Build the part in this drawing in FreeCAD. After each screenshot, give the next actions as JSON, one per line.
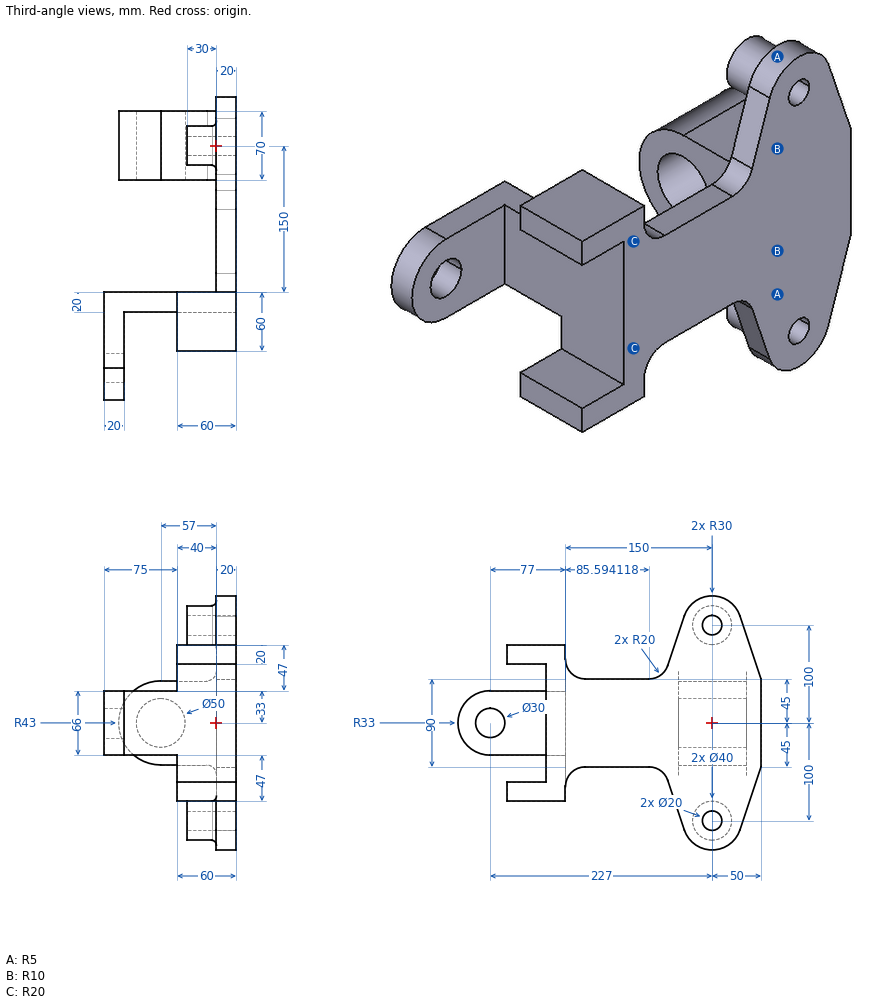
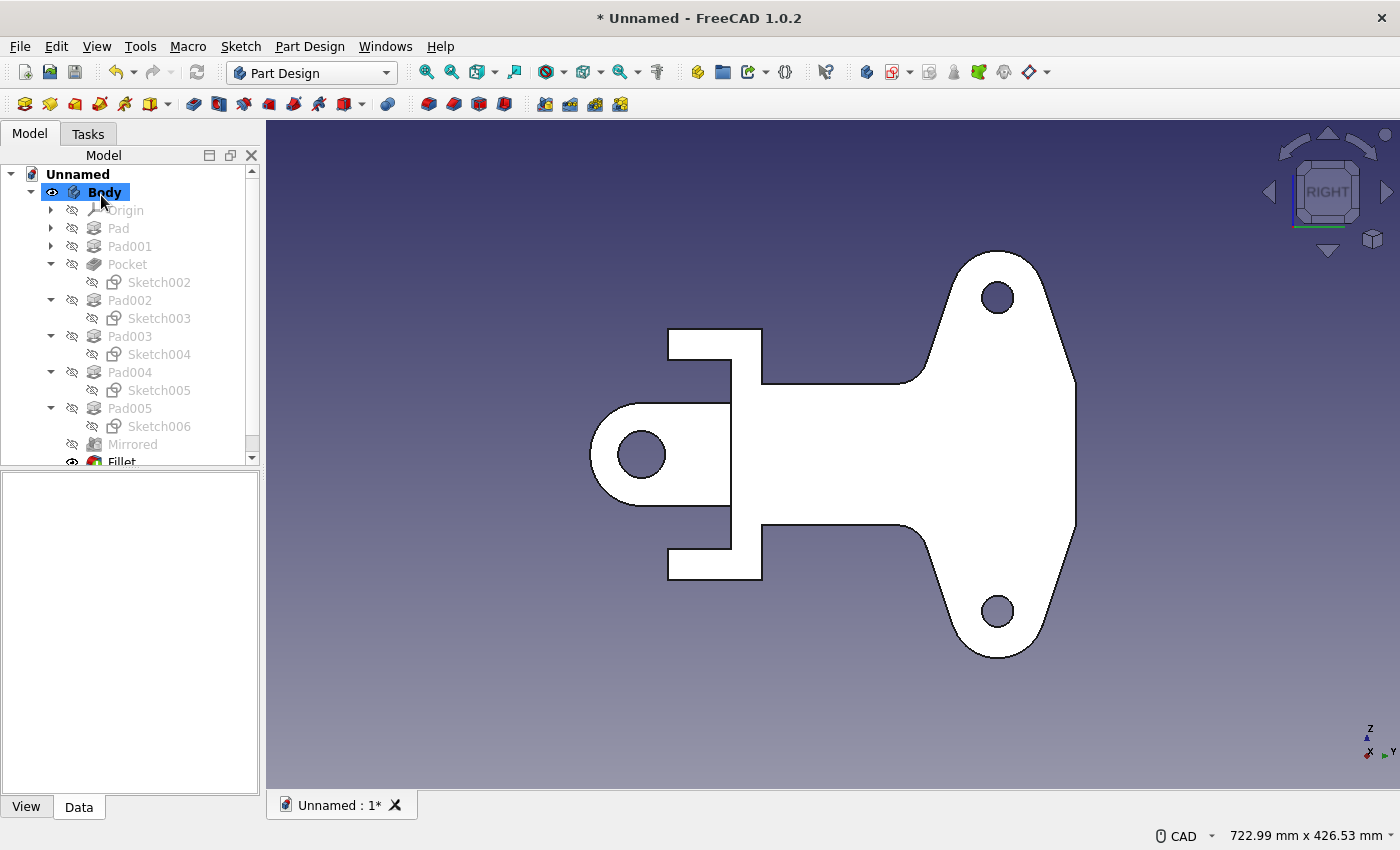
{"action": "key", "text": "5"}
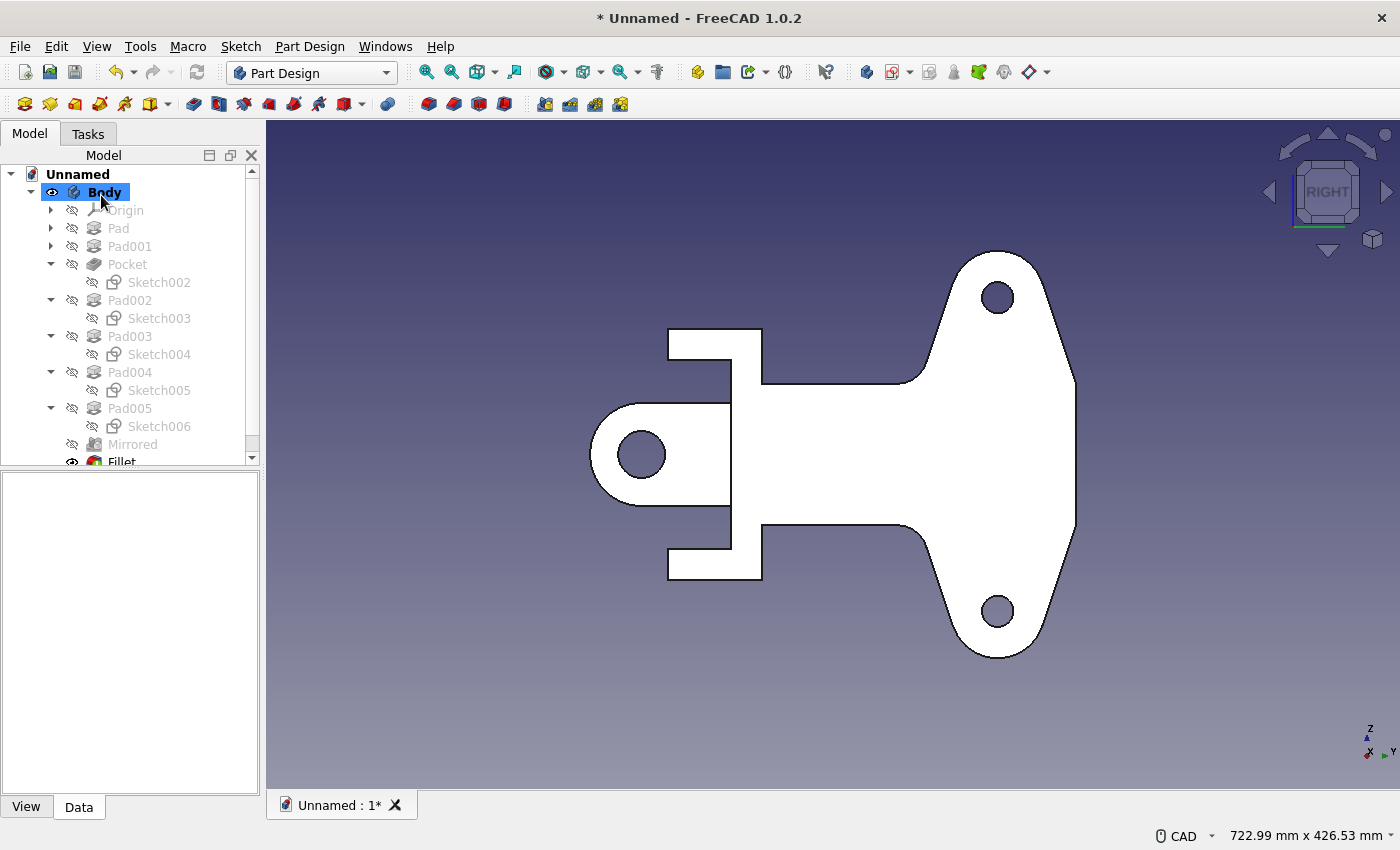
{"action": "key", "text": "4"}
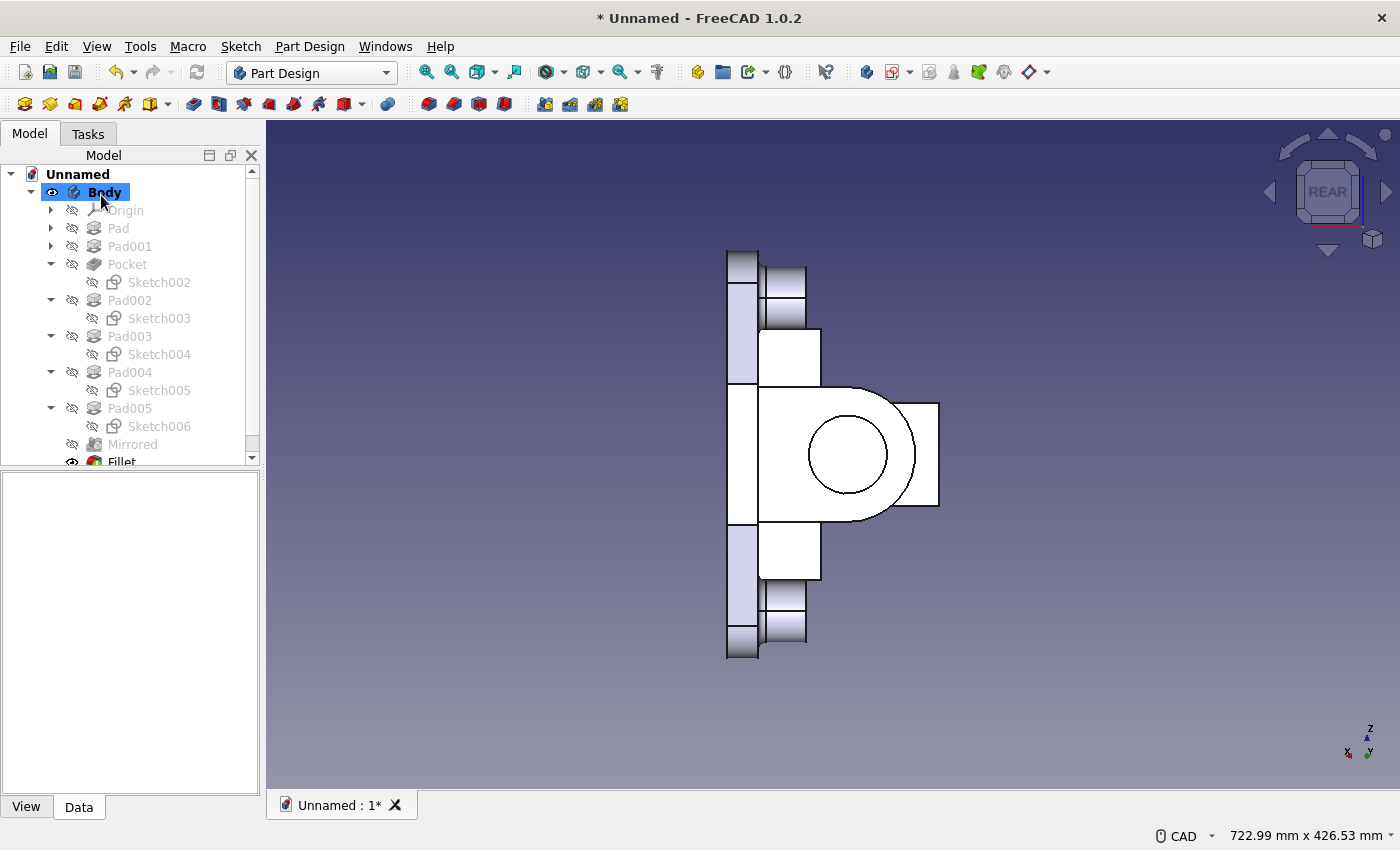
{"action": "key", "text": "6"}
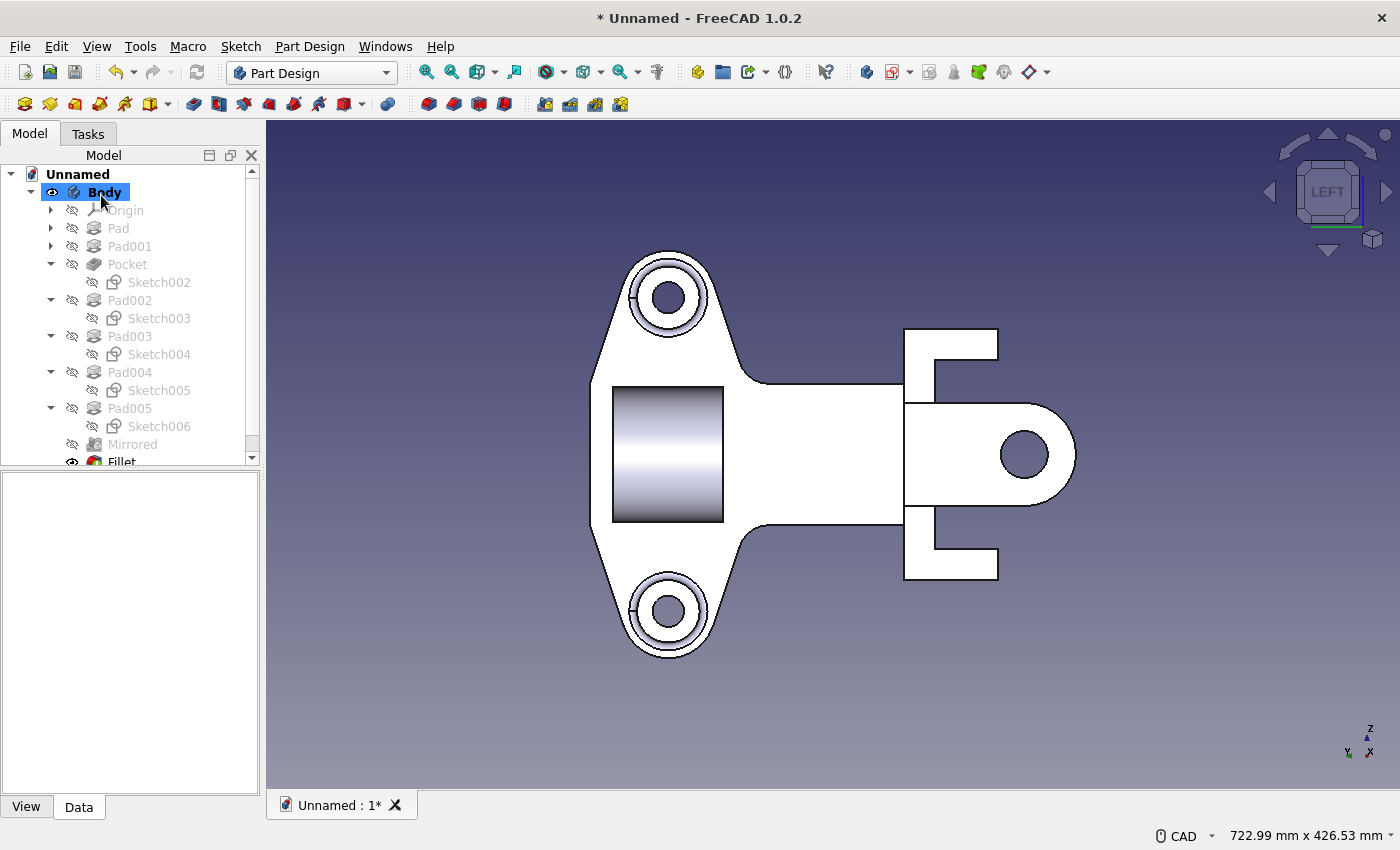
{"action": "key", "text": "v 3"}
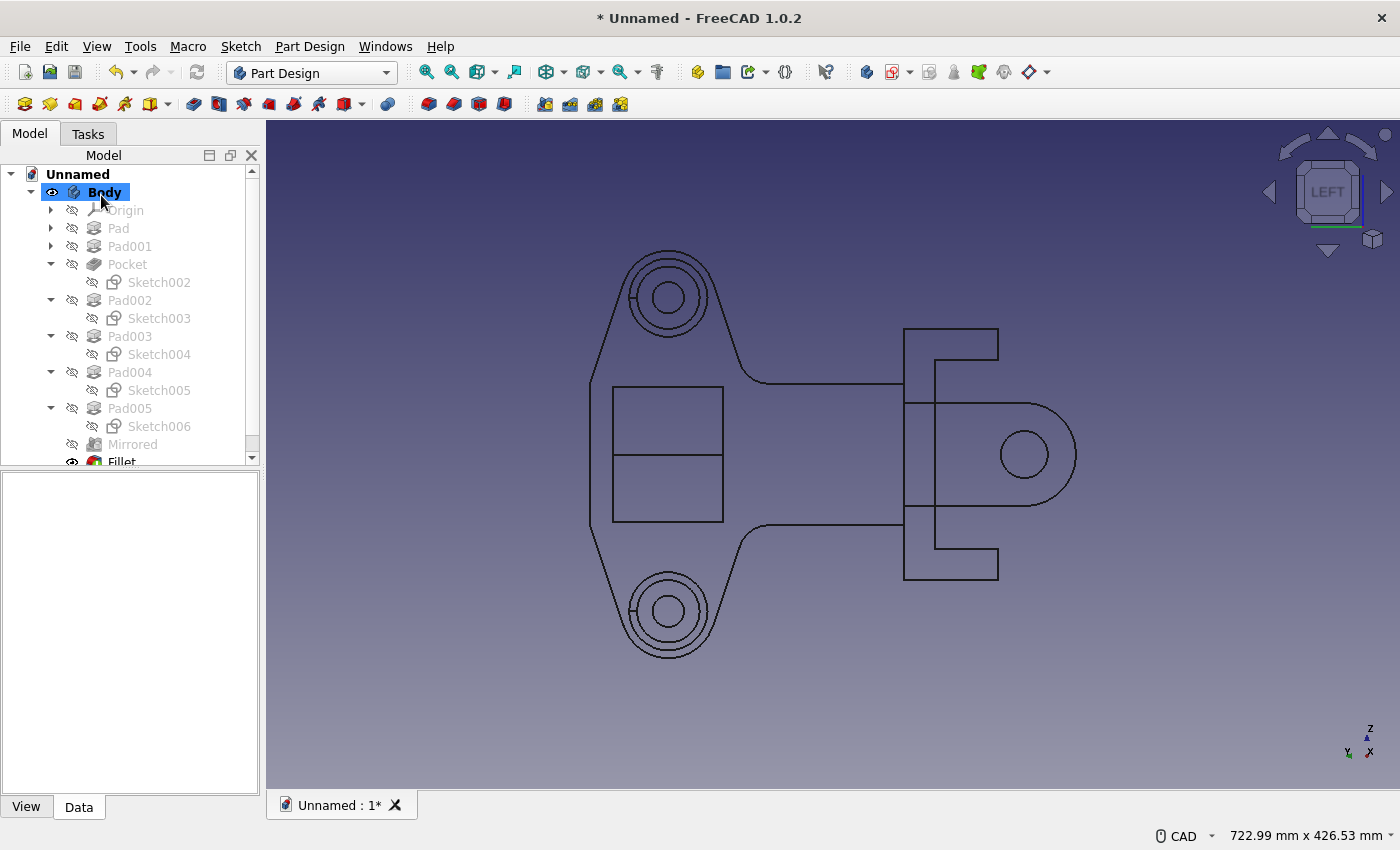
{"action": "key", "text": "0"}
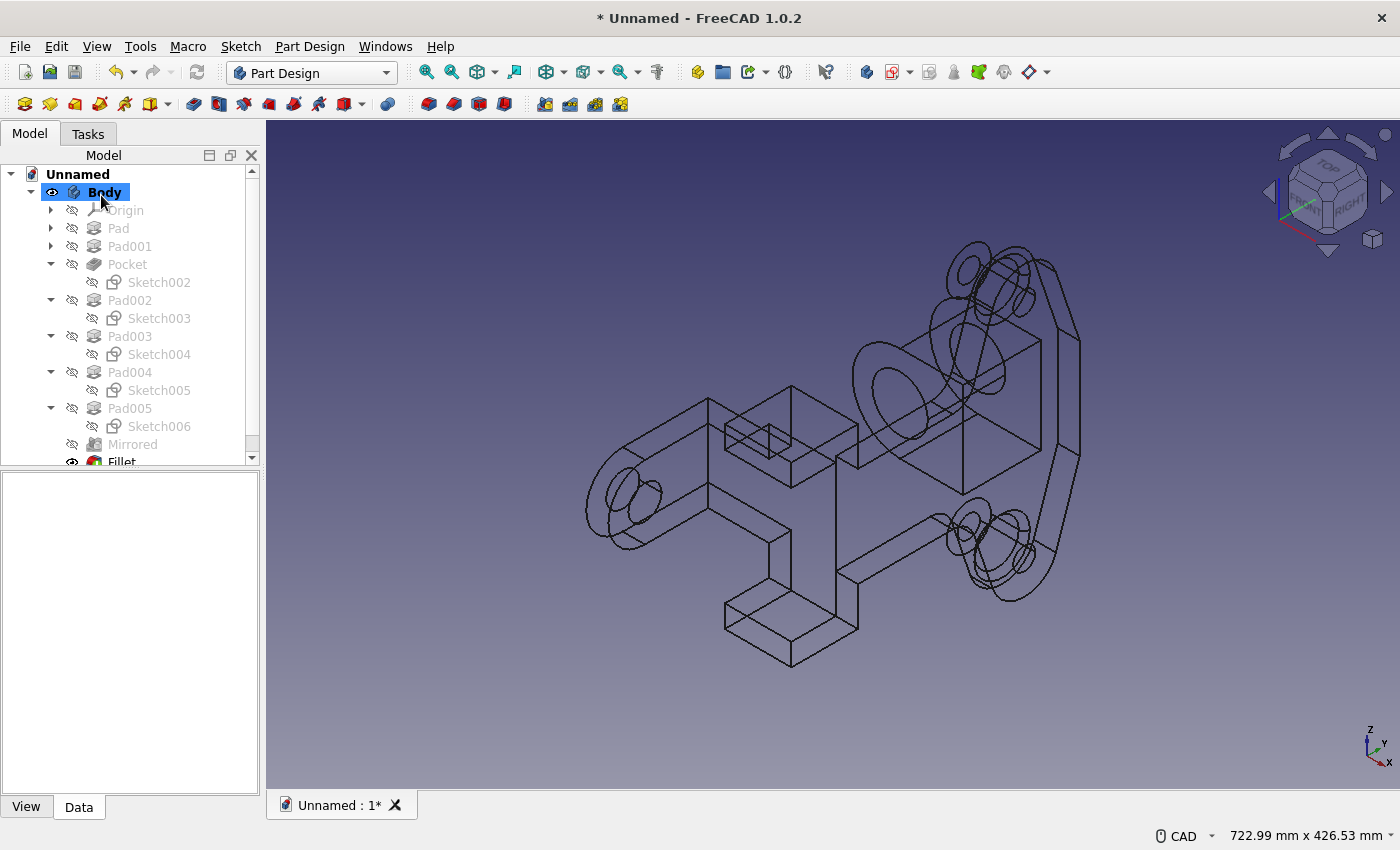
{"action": "left_click", "coordinate": [1002, 362]}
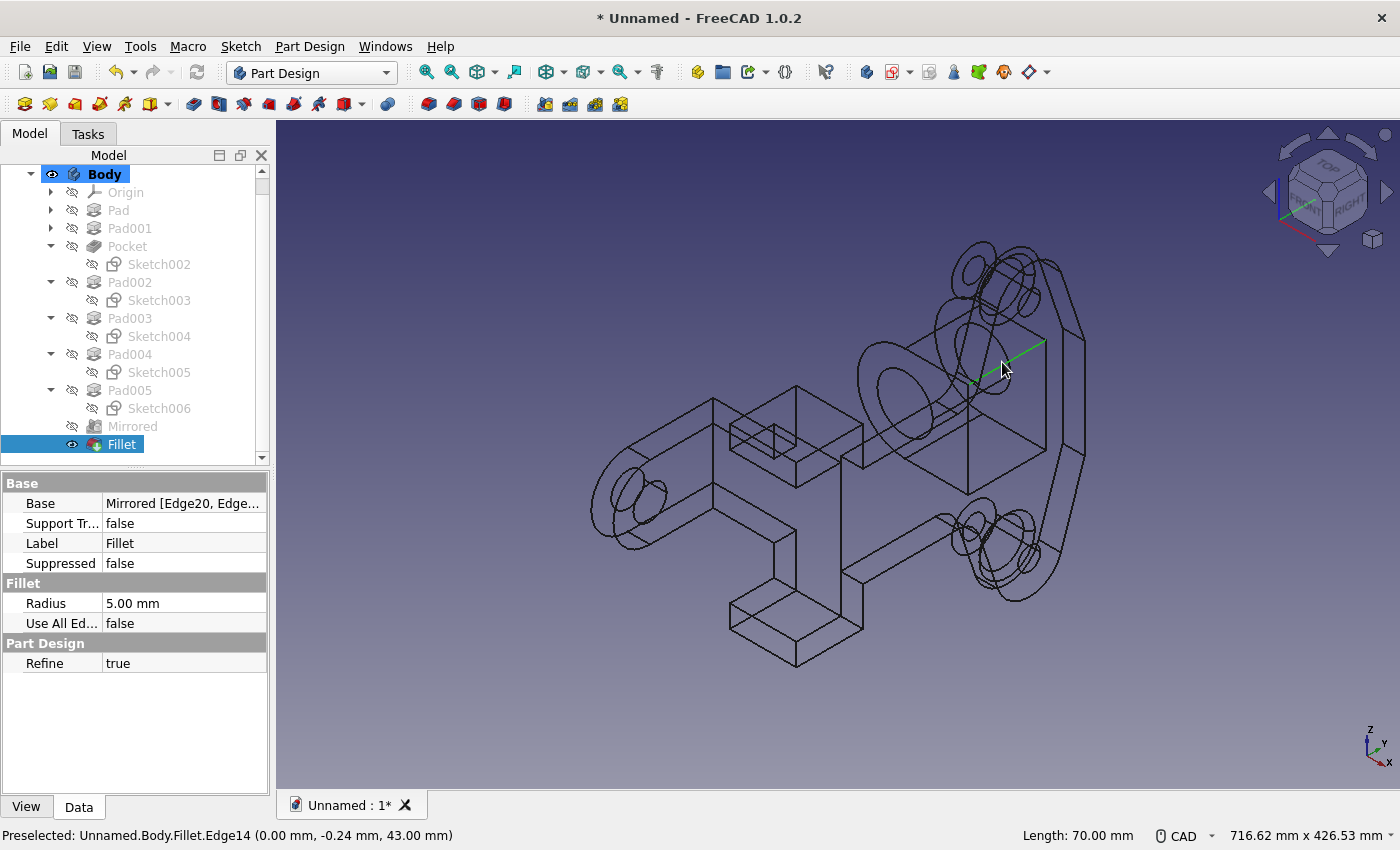
{"action": "left_click", "coordinate": [1007, 472], "text": "ctrl"}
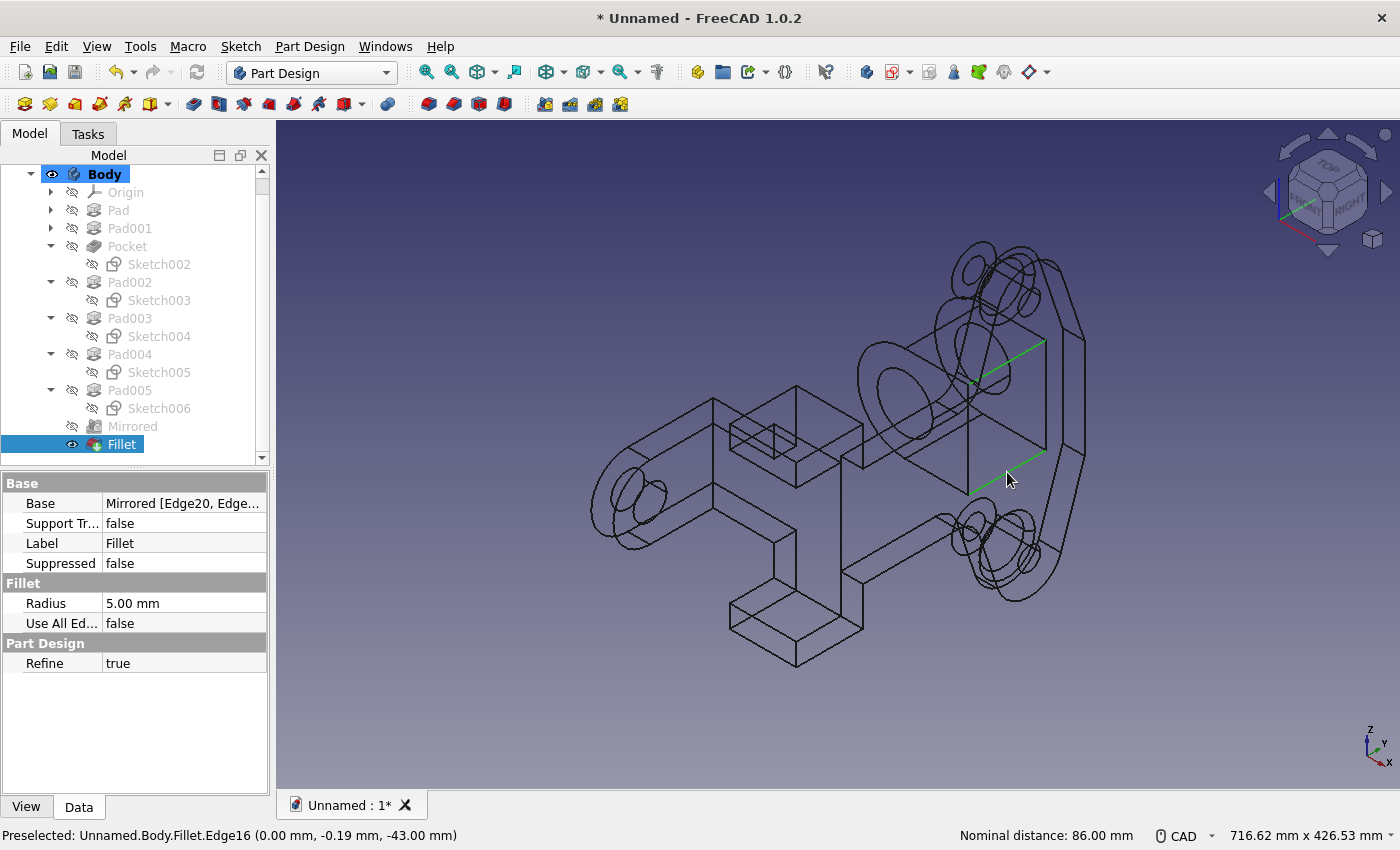
{"action": "key", "text": "v 1"}